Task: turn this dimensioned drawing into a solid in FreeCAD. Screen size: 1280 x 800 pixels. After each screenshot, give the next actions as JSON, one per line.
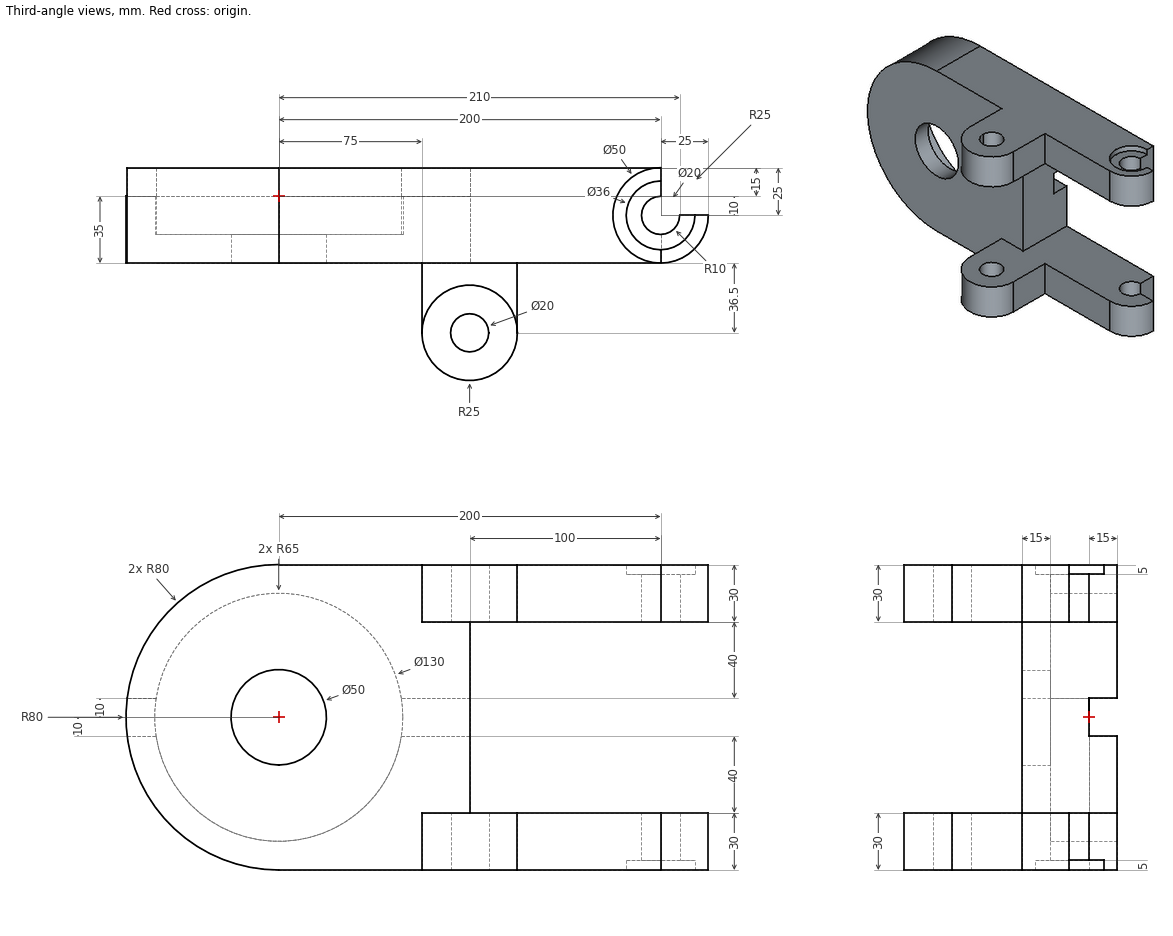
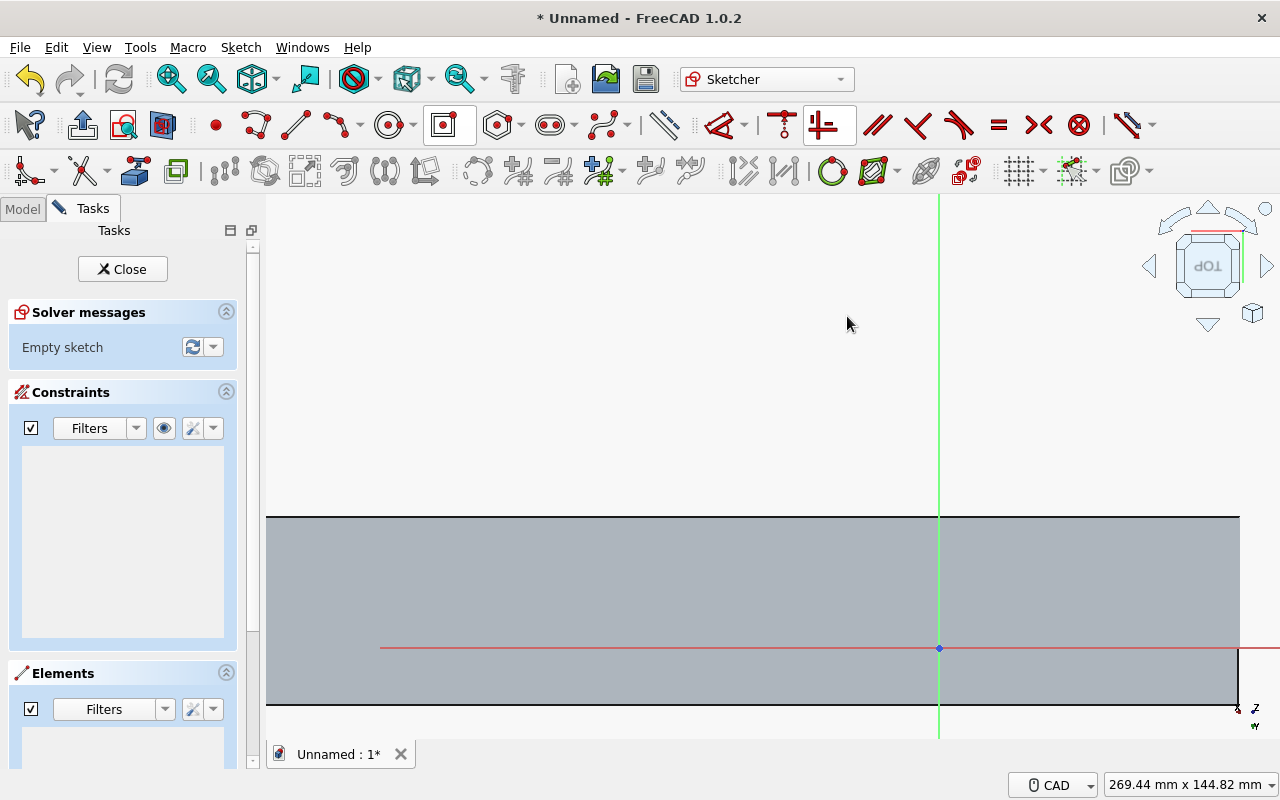
{"action": "left_click", "coordinate": [256, 126]}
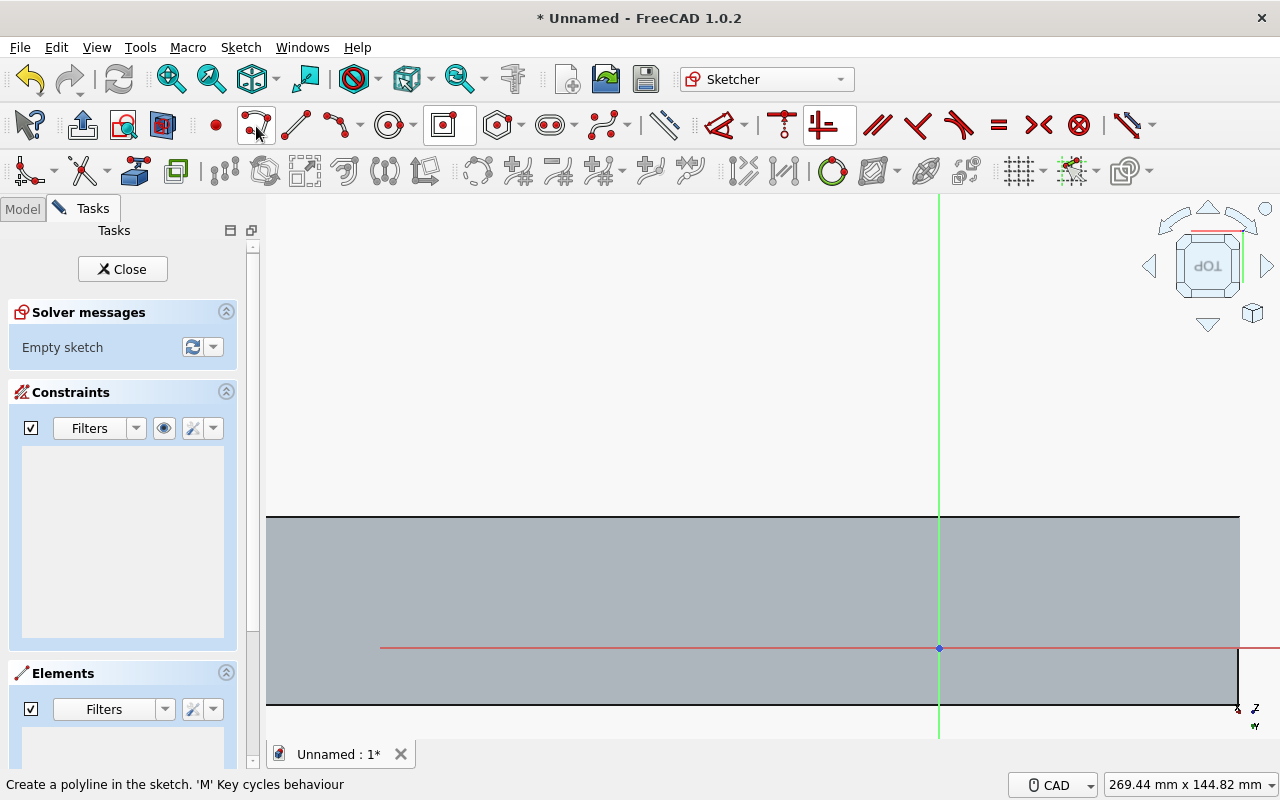
{"action": "left_click", "coordinate": [469, 379]}
{"action": "left_click", "coordinate": [469, 517]}
{"action": "left_click", "coordinate": [657, 517]}
{"action": "left_click", "coordinate": [657, 379]}
{"action": "right_click", "coordinate": [657, 379]}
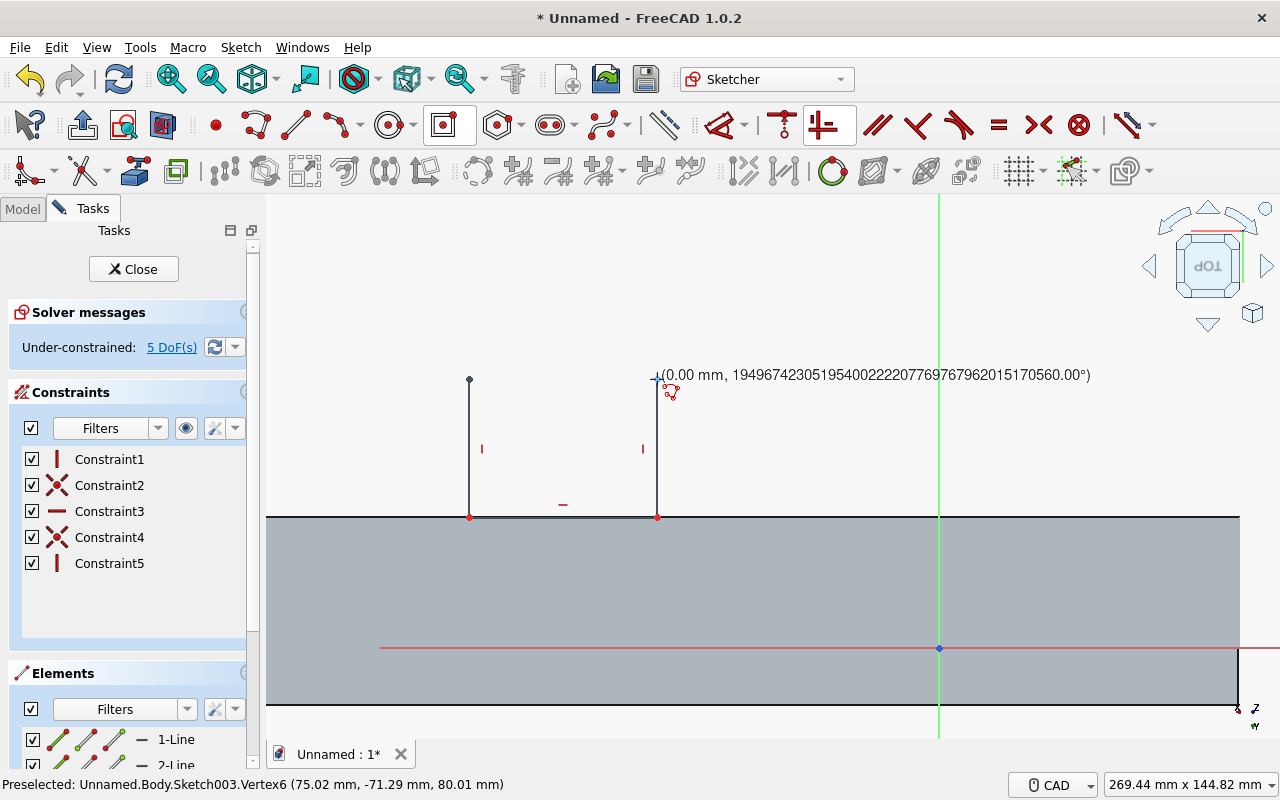
{"action": "key", "text": "g 3 a"}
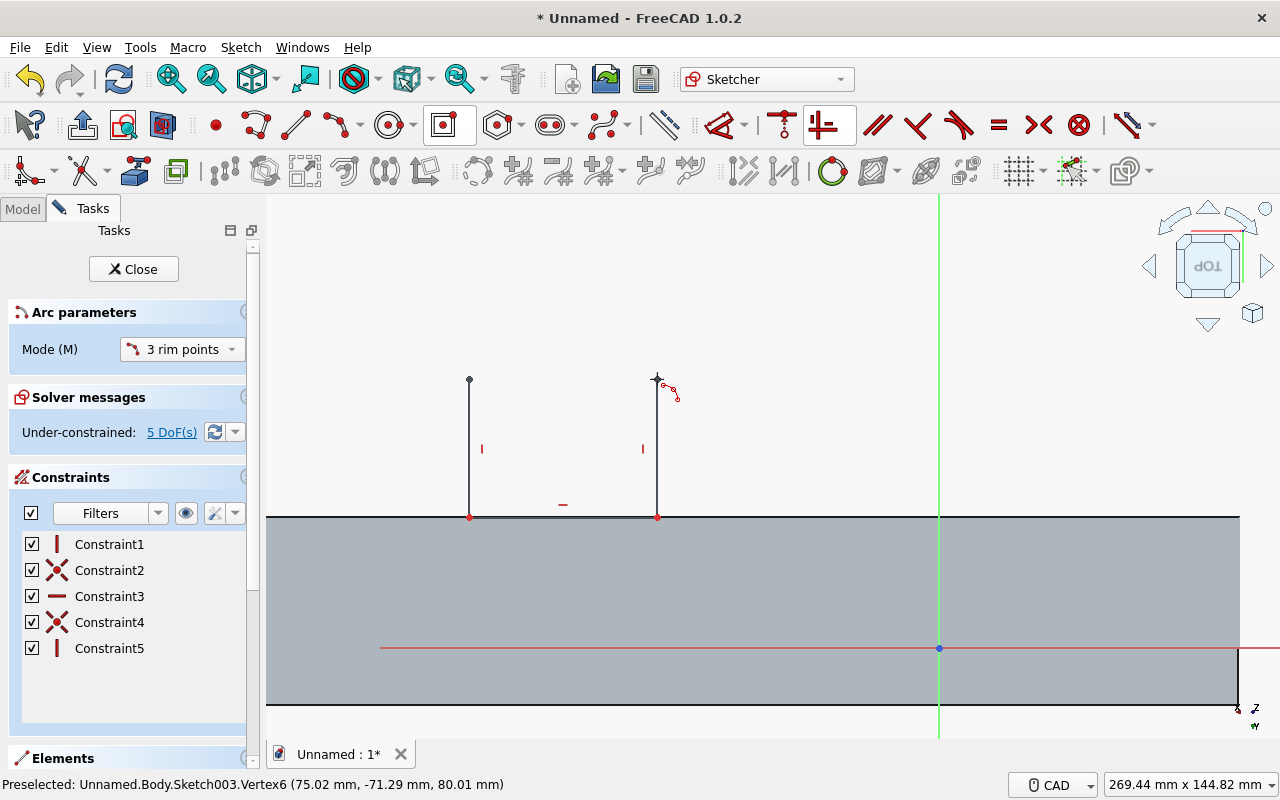
{"action": "left_click", "coordinate": [657, 380]}
{"action": "left_click", "coordinate": [469, 380]}
{"action": "left_click", "coordinate": [563, 285]}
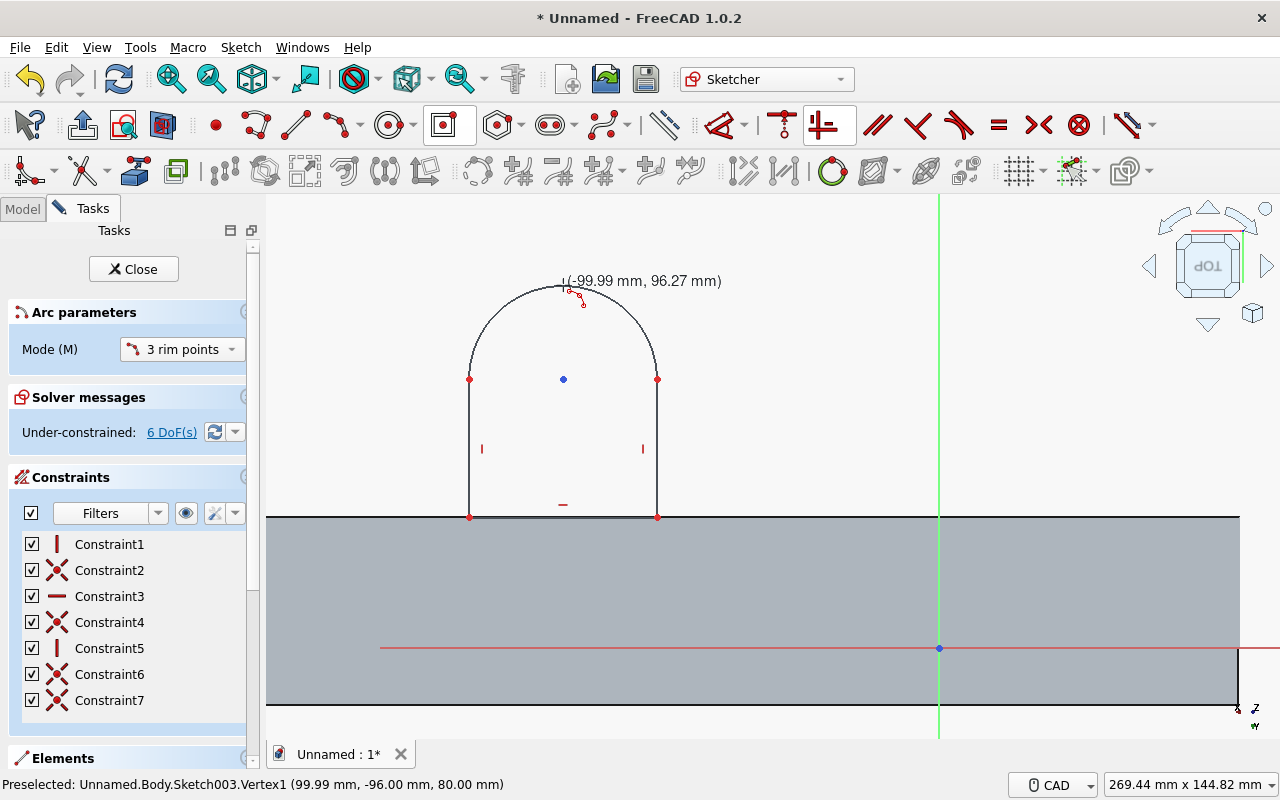
{"action": "left_click", "coordinate": [390, 126]}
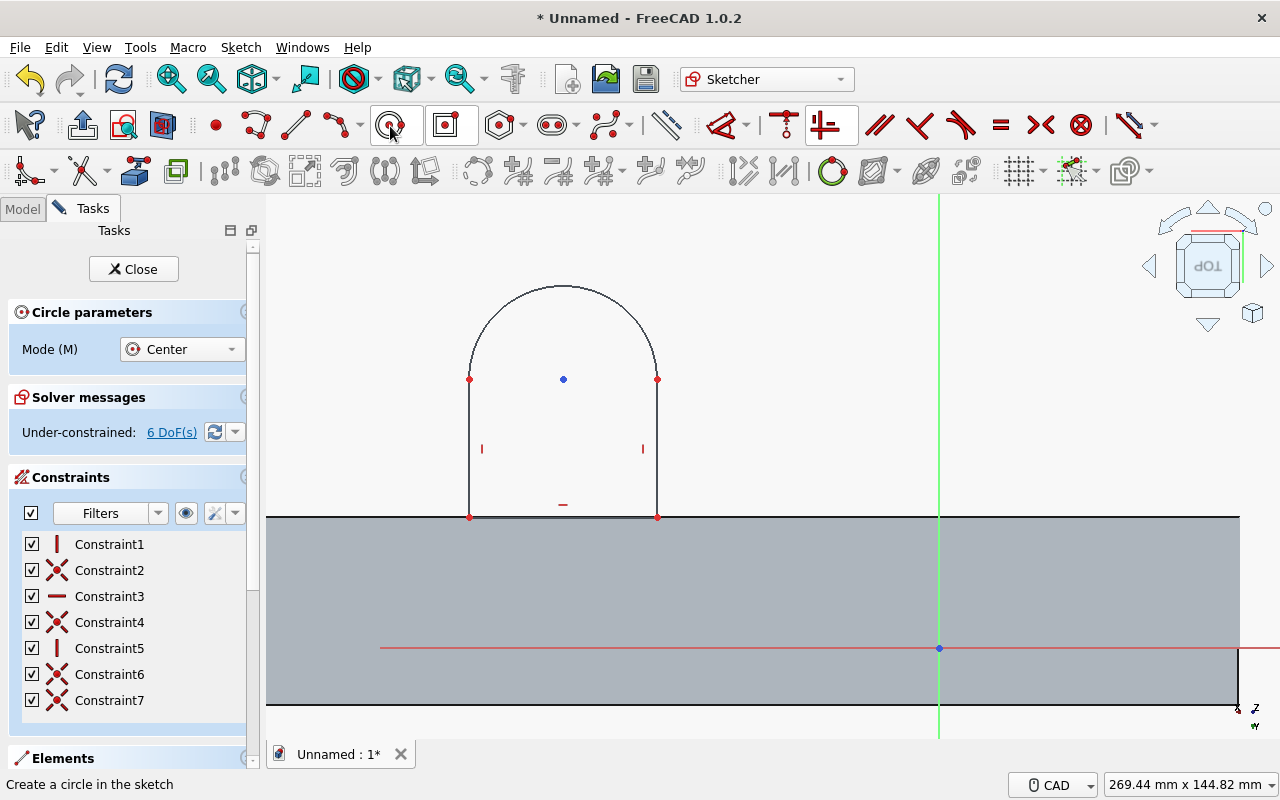
{"action": "left_click", "coordinate": [563, 379]}
{"action": "left_click", "coordinate": [590, 353]}
{"action": "key", "text": "Escape"}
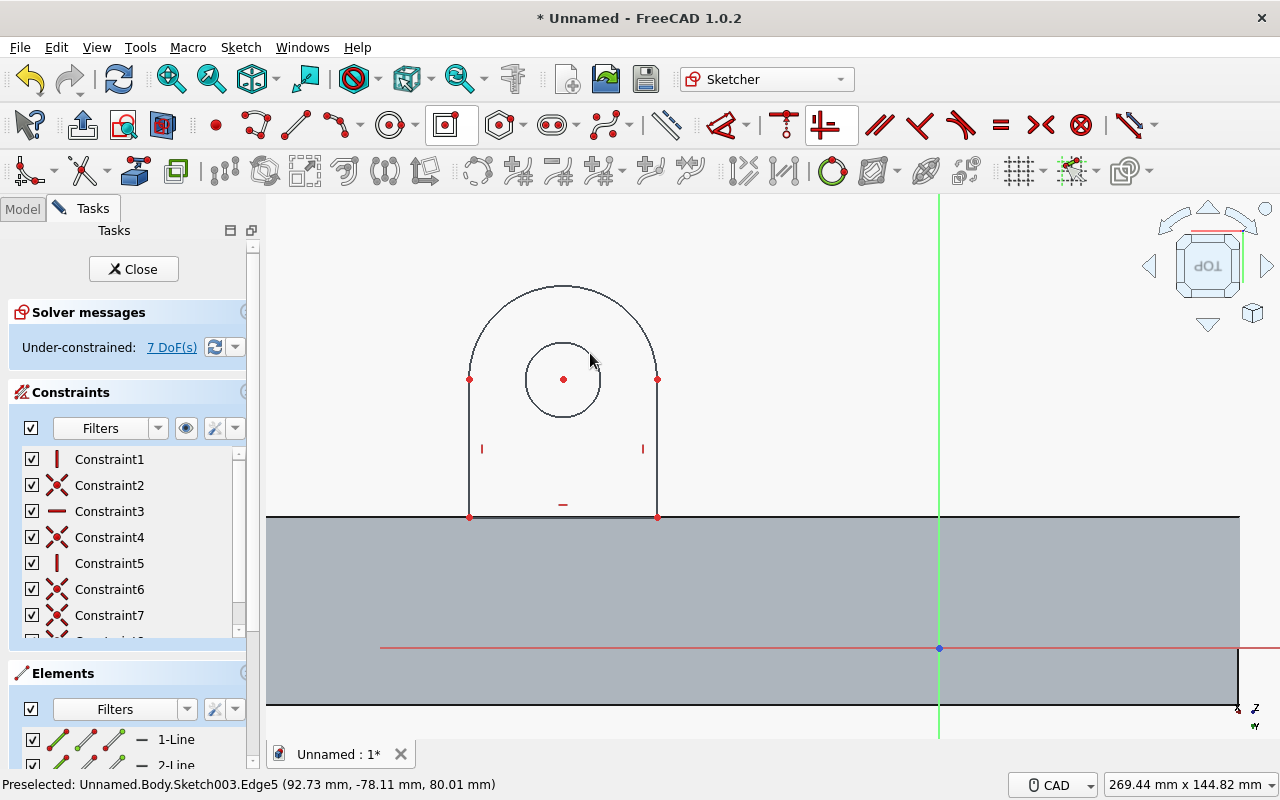
{"action": "left_click", "coordinate": [469, 421]}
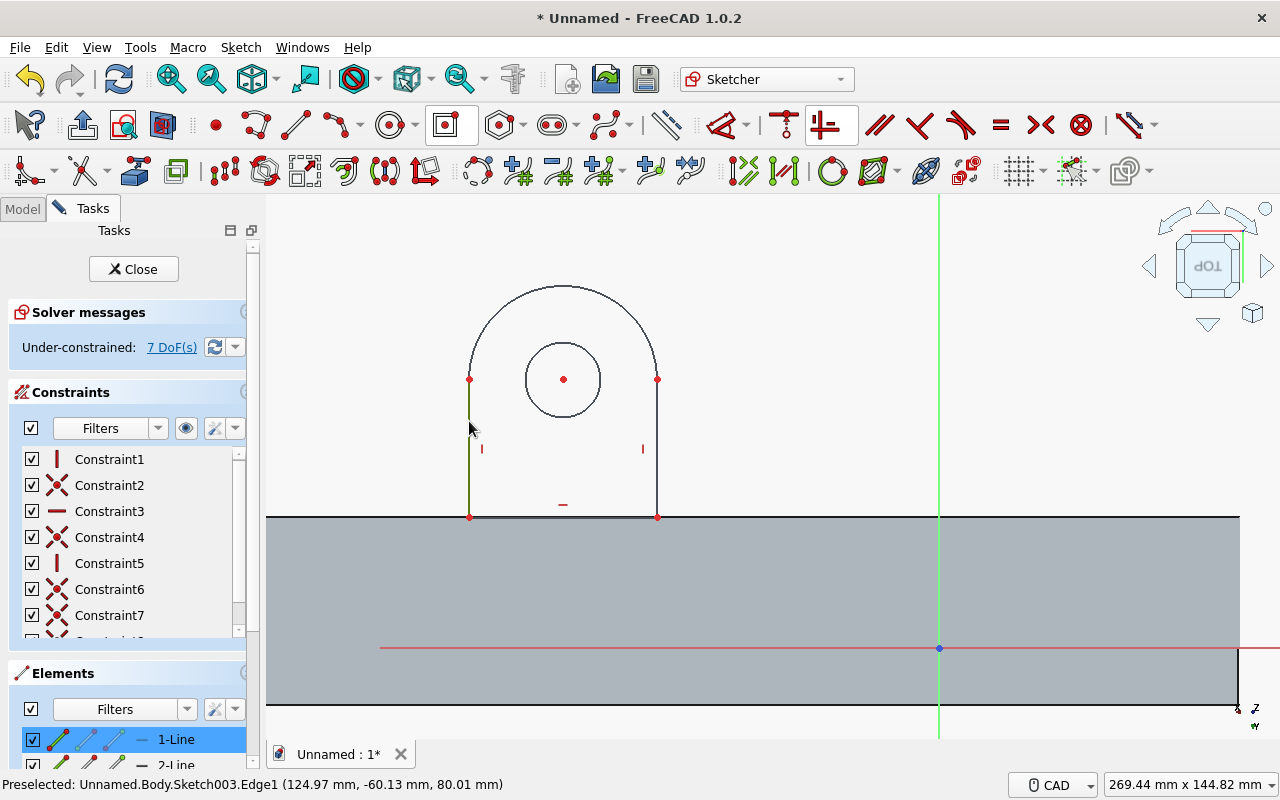
{"action": "left_click", "coordinate": [618, 304]}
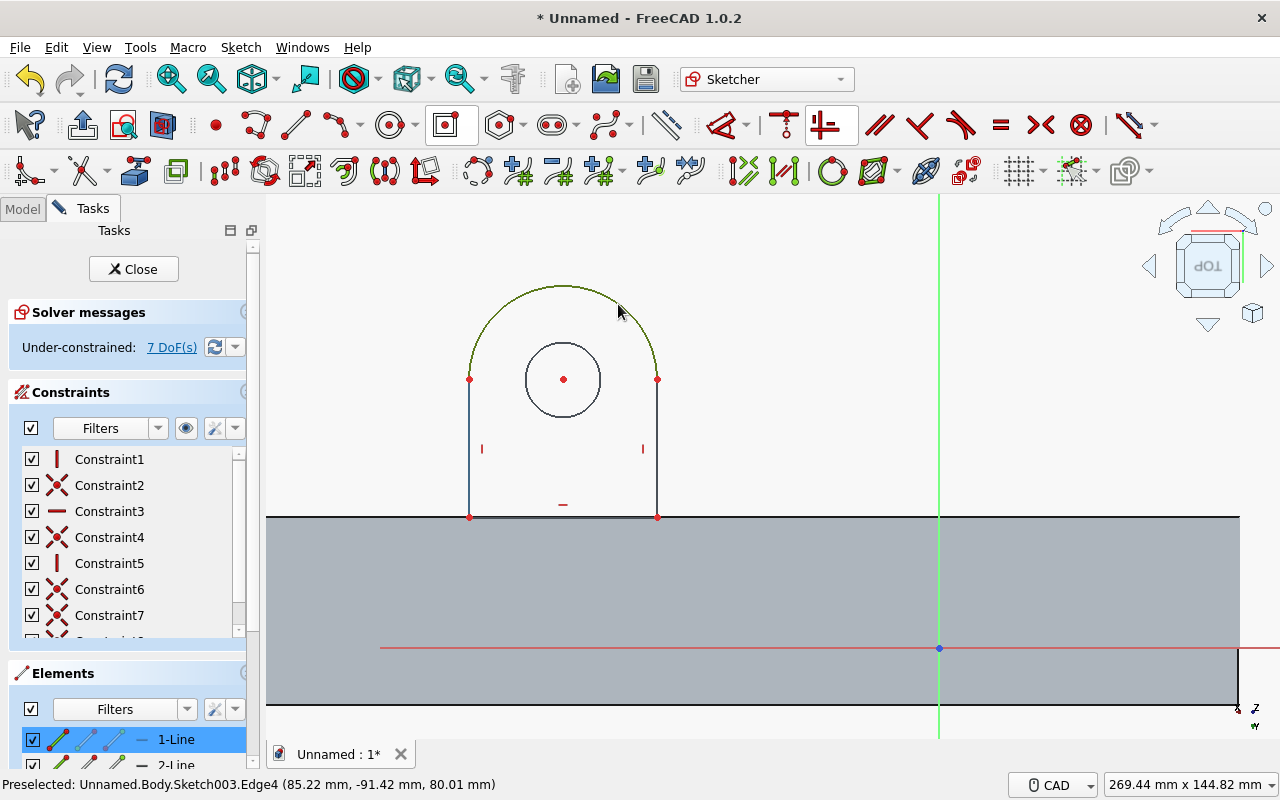
{"action": "left_click", "coordinate": [962, 126]}